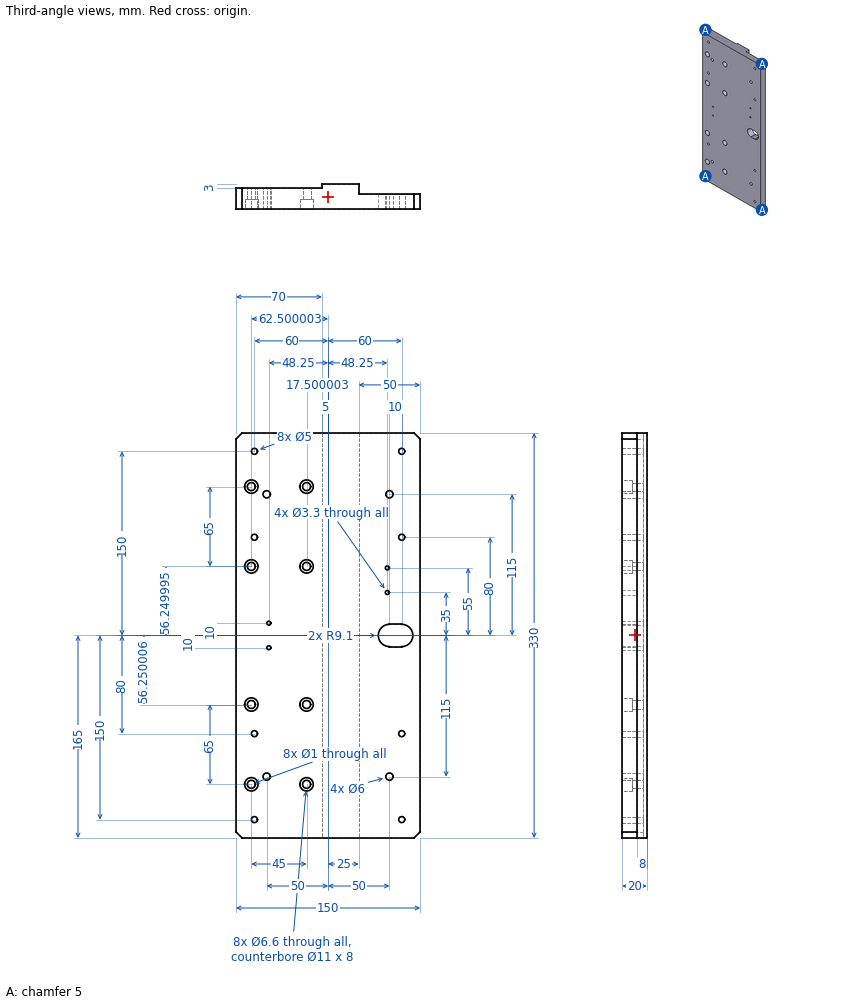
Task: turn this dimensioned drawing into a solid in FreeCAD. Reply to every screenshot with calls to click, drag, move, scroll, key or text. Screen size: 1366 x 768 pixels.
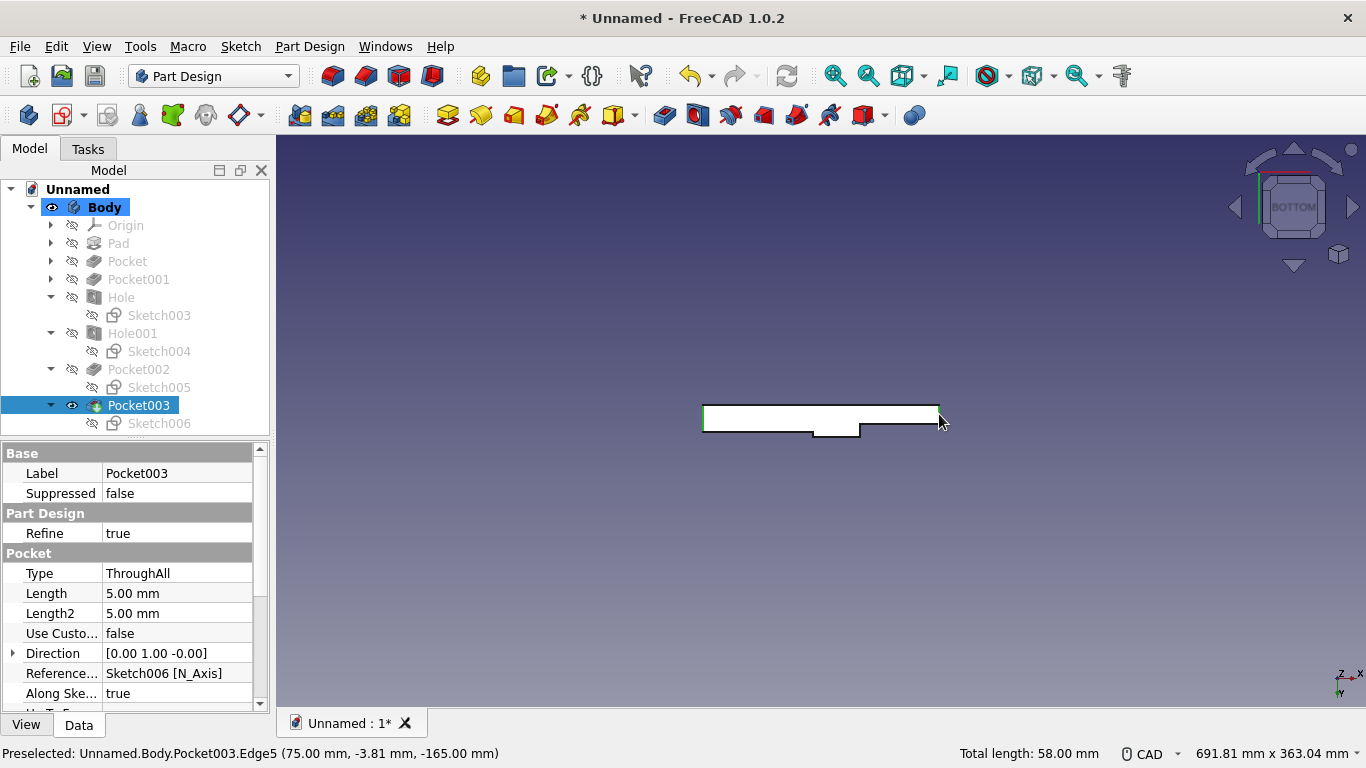
click(366, 76)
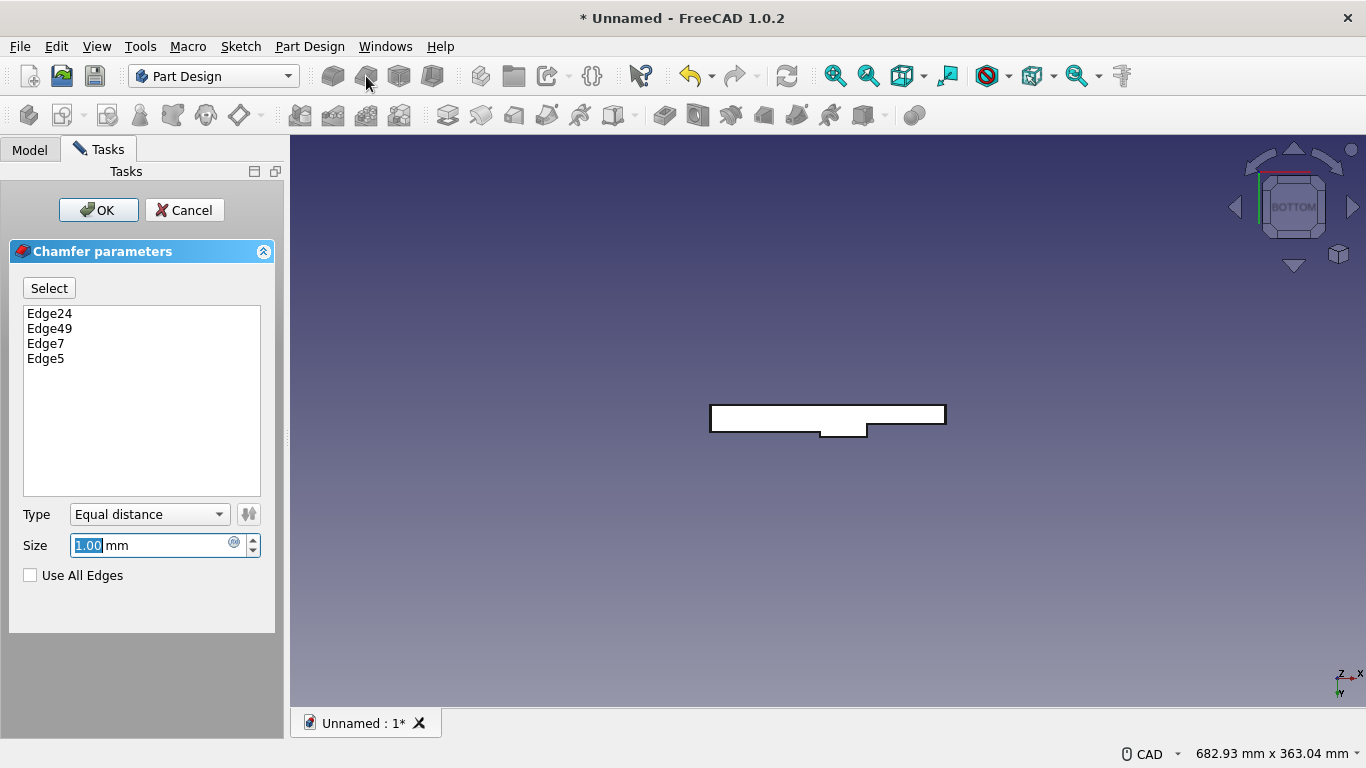
text(5)
key(Tab)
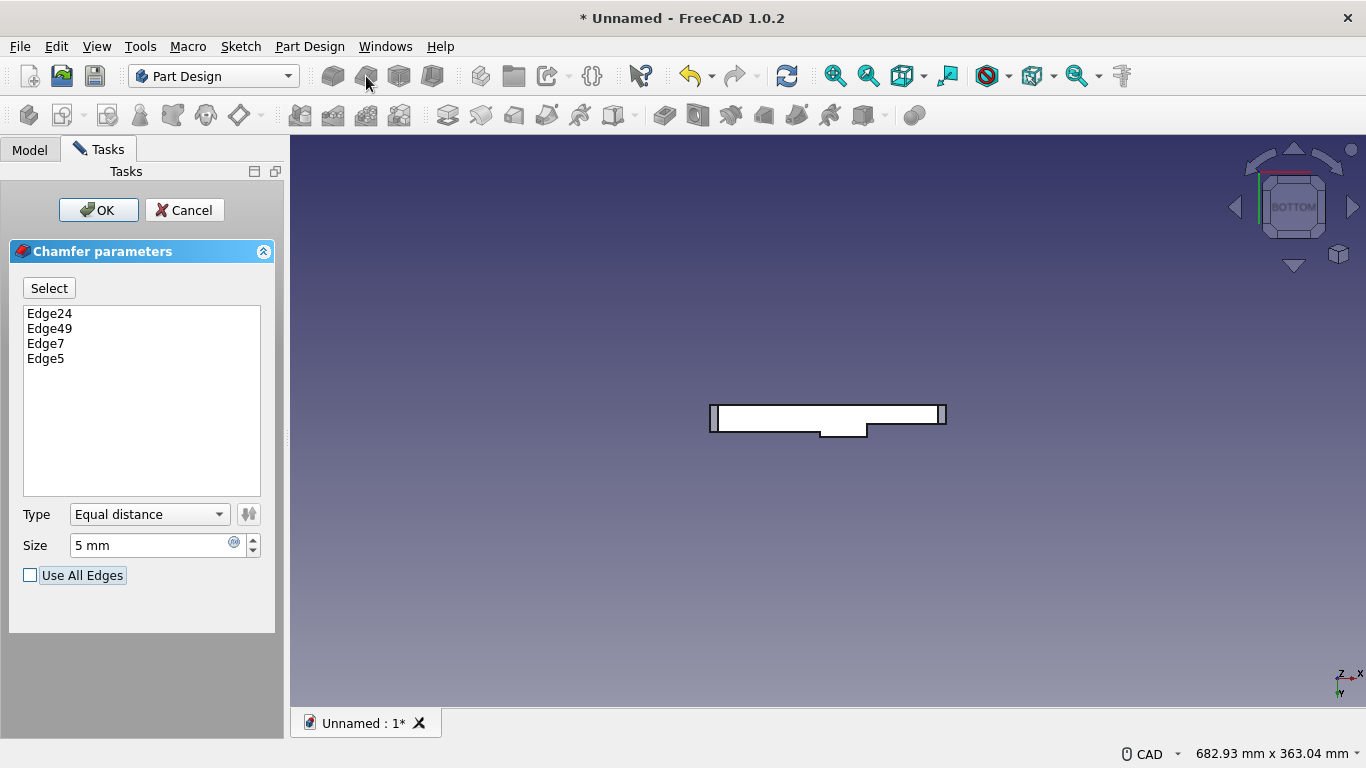
click(99, 210)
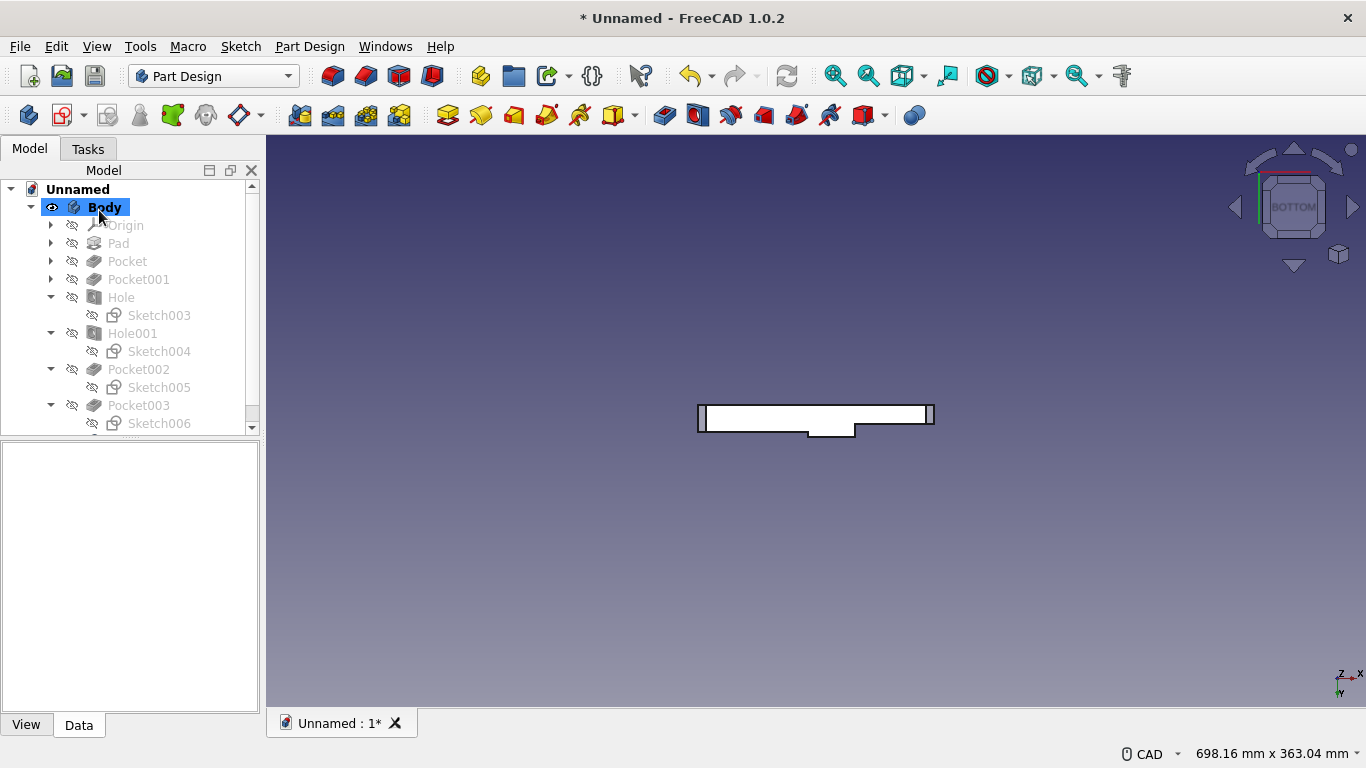
click(836, 76)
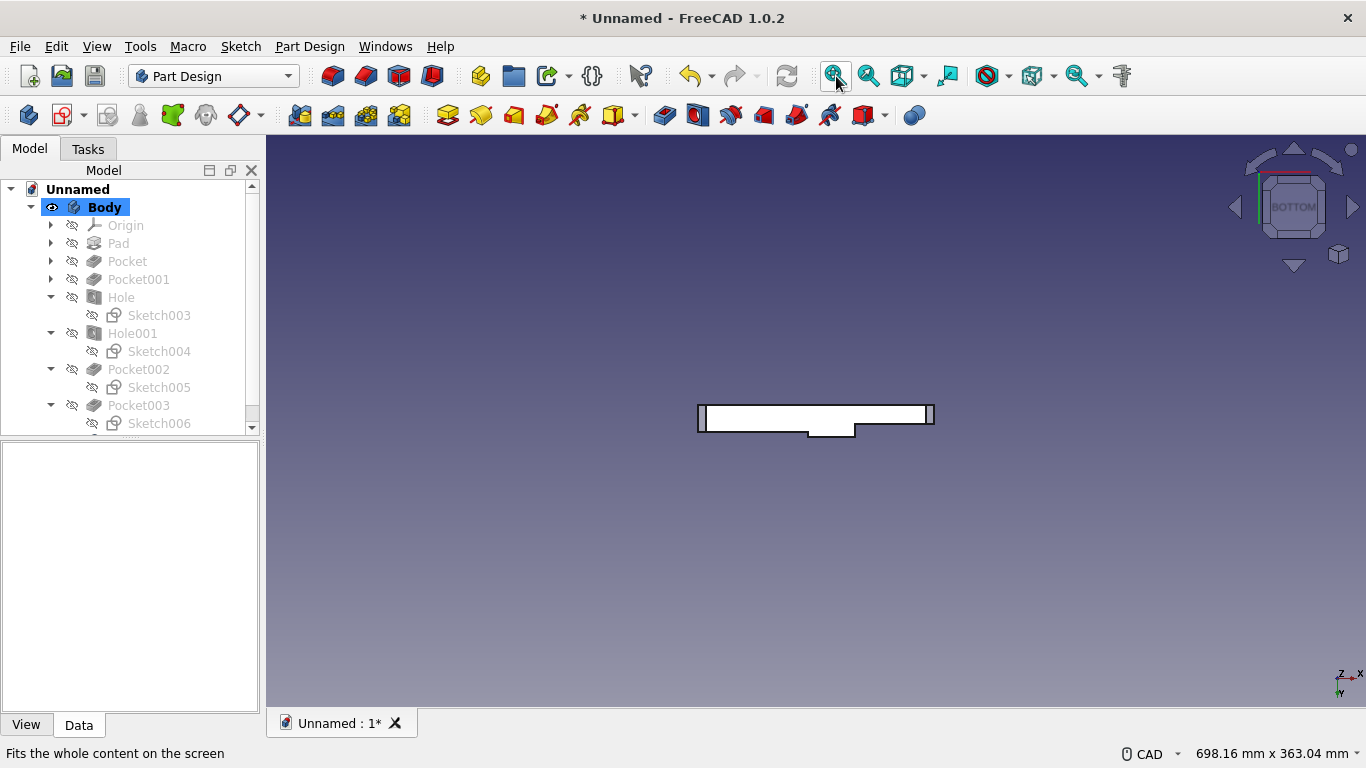
key(0)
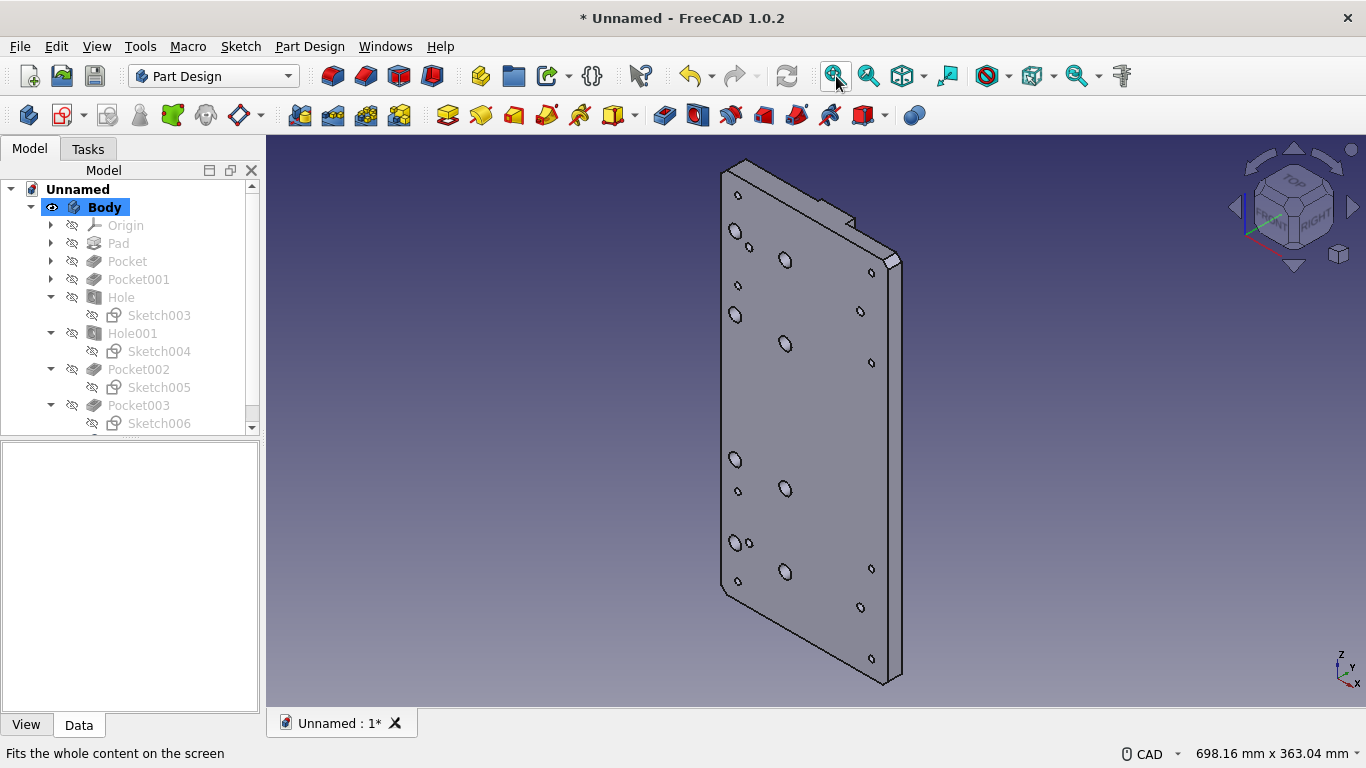
click(829, 440)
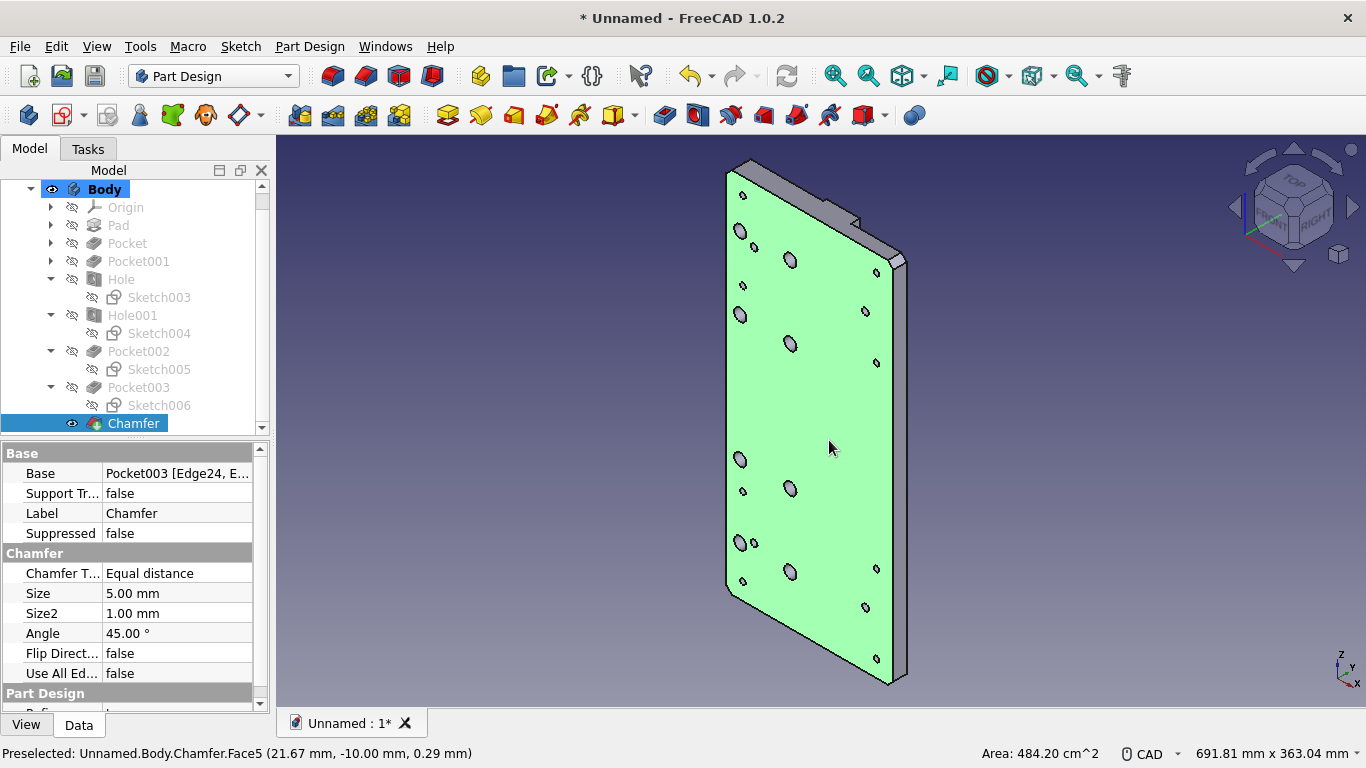
click(62, 116)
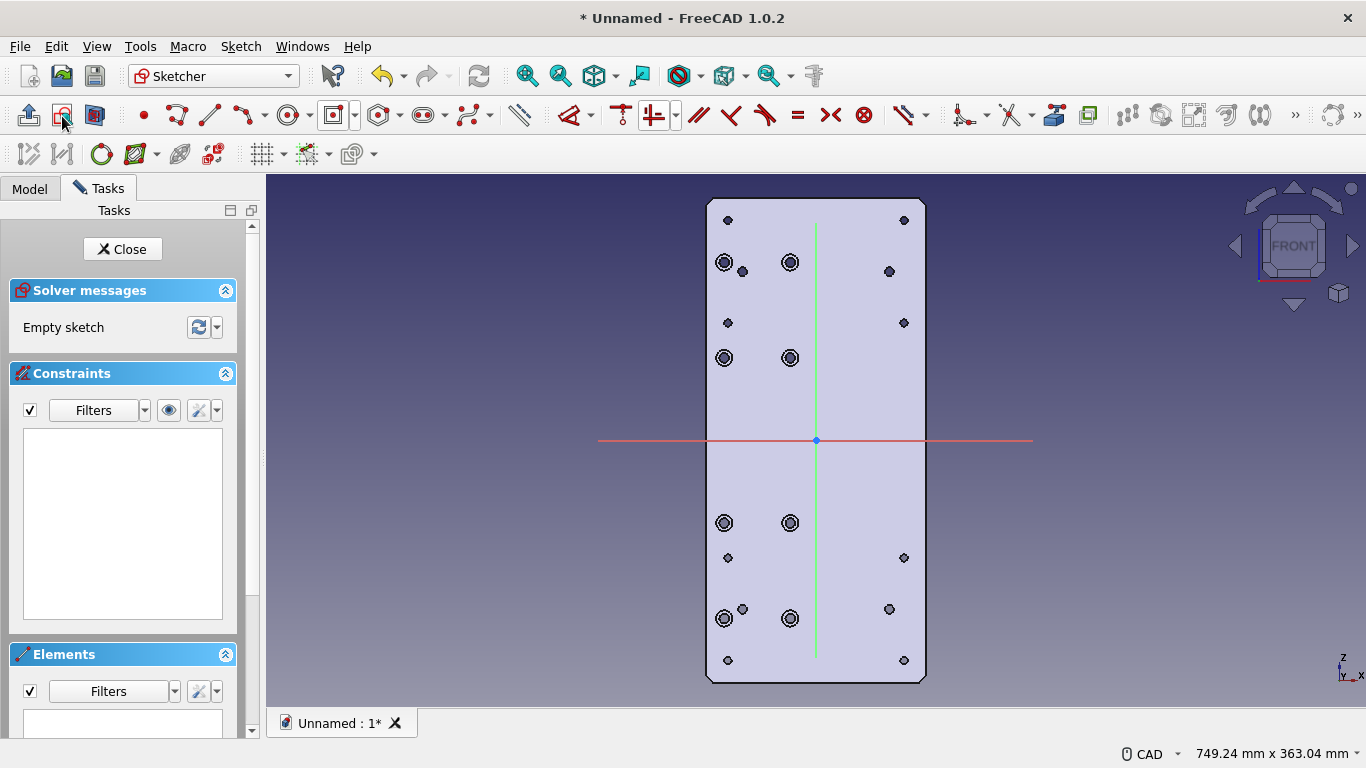
scroll(890, 440, up, 9)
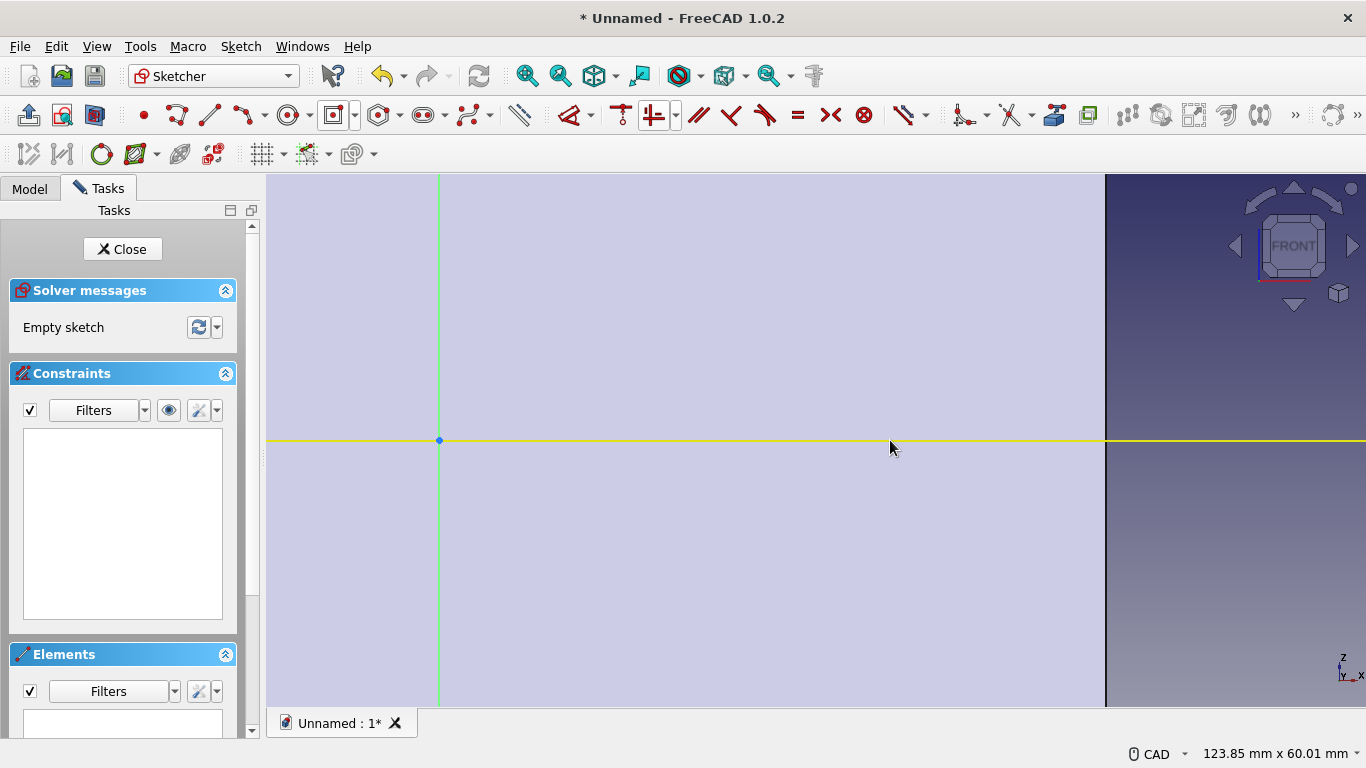
click(422, 116)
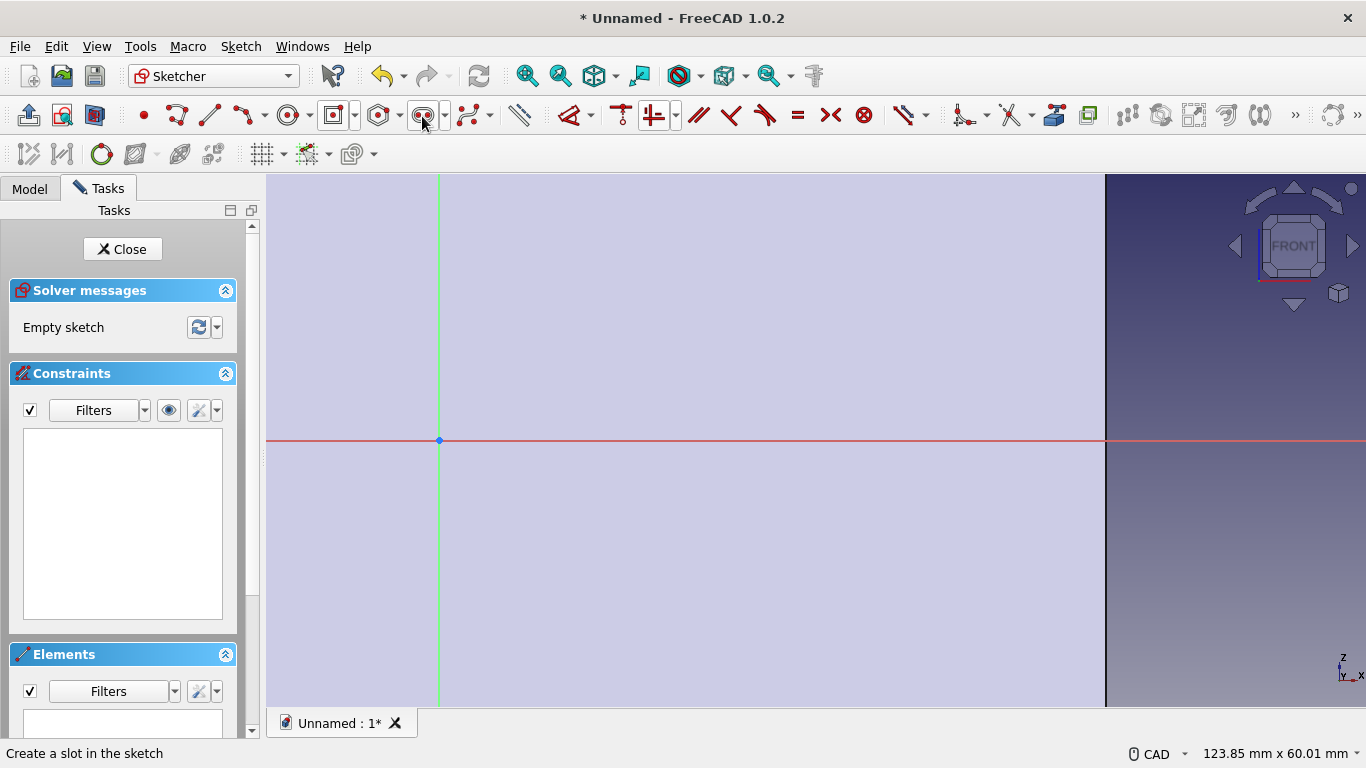
click(884, 440)